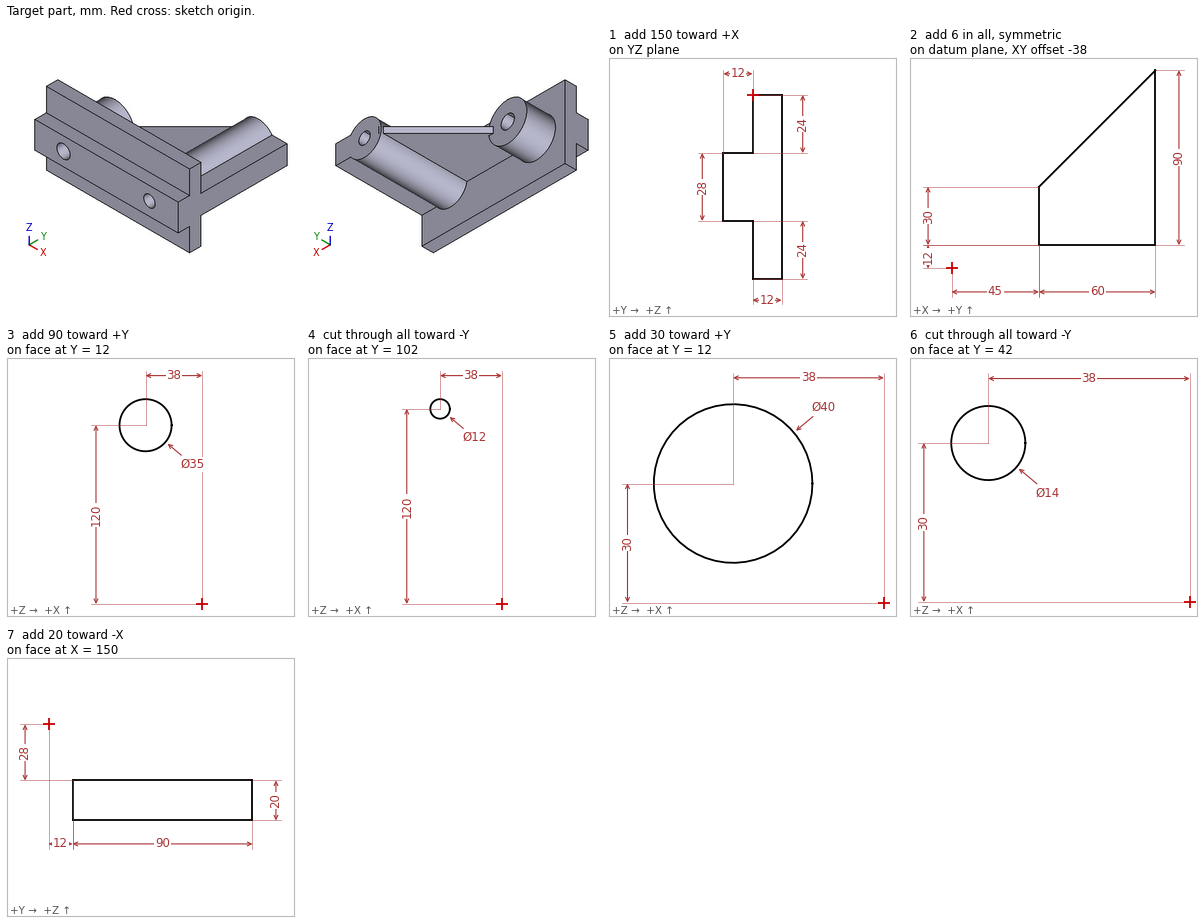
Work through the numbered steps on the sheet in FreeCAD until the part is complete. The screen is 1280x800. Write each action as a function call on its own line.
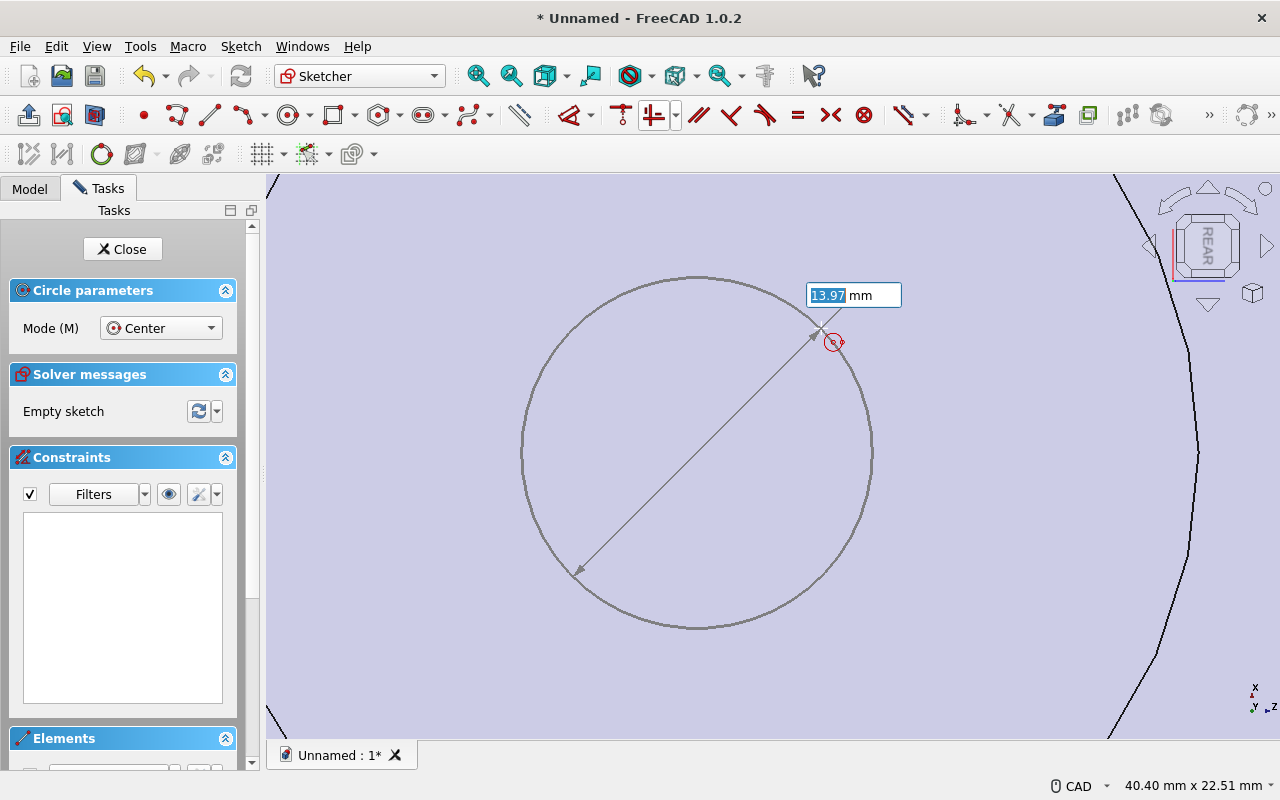
text(14)
key(Return)
key(Escape)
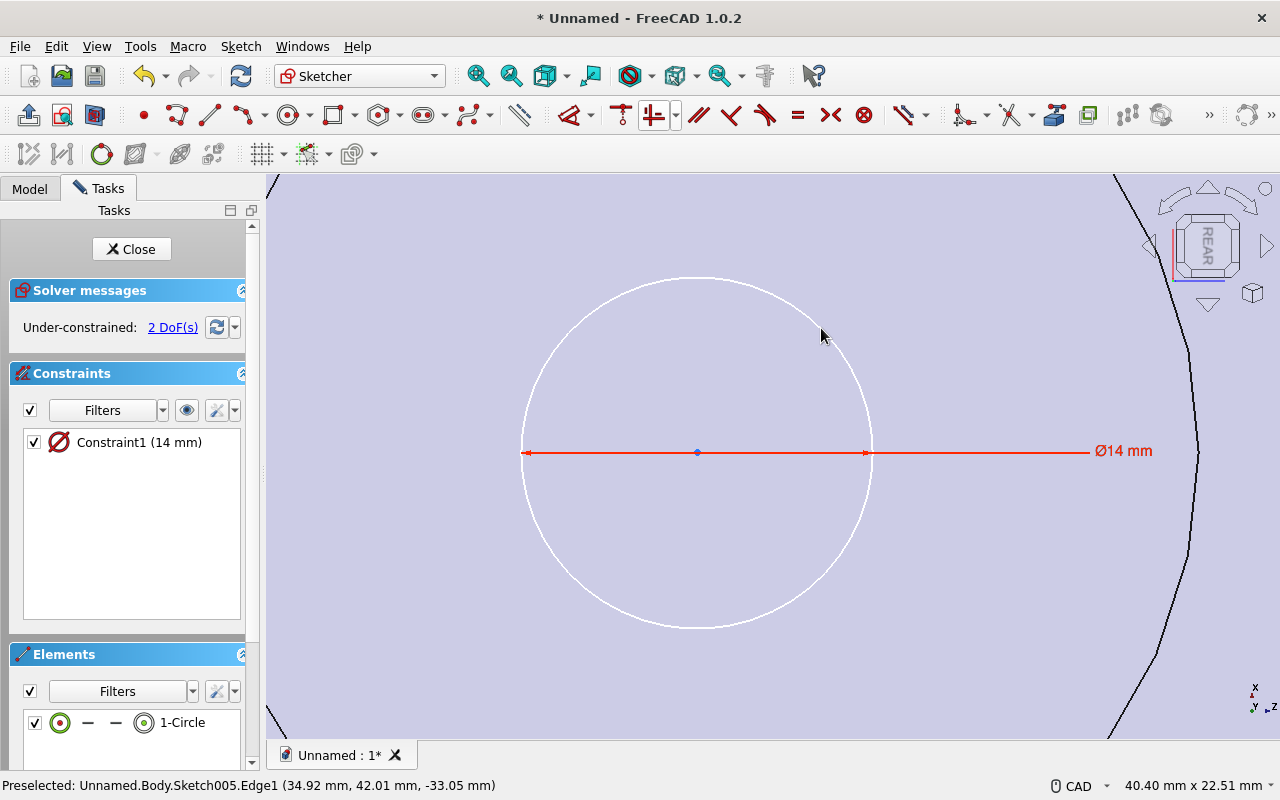
click(568, 116)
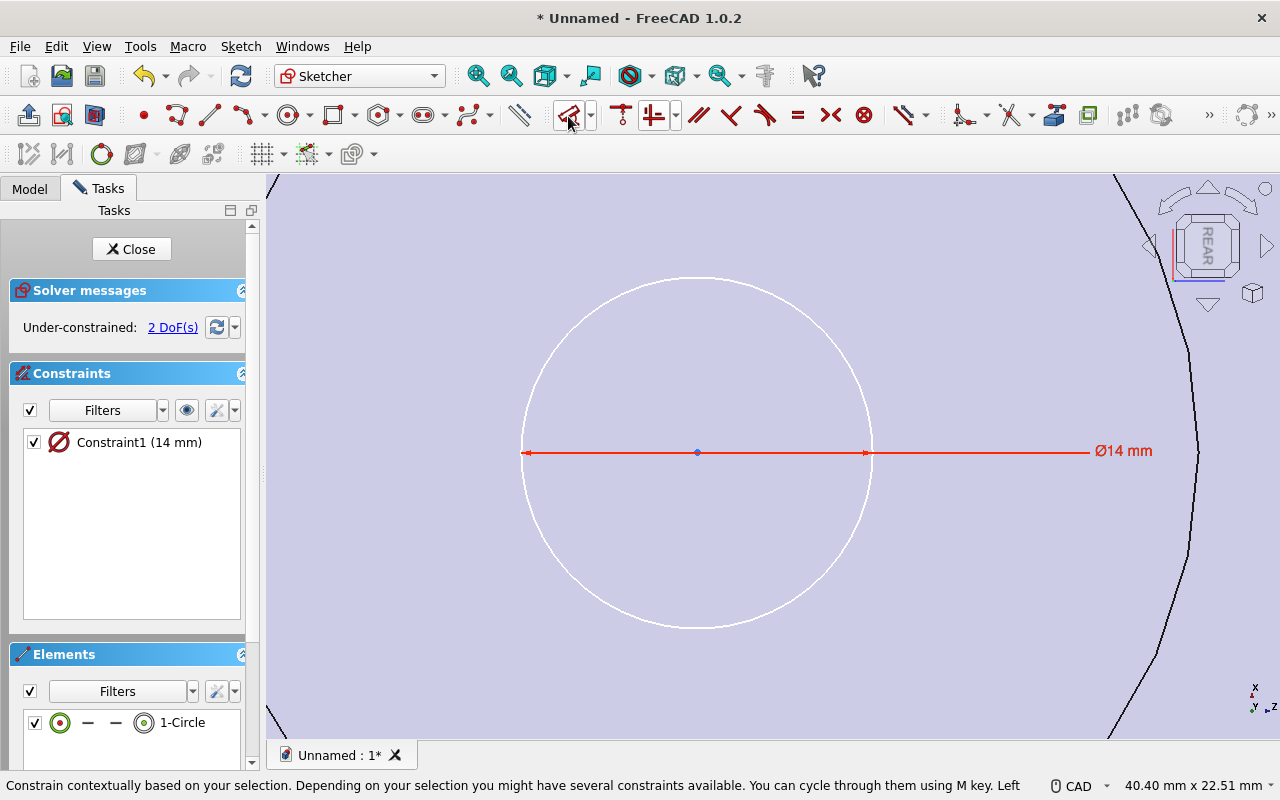
click(697, 453)
click(906, 419)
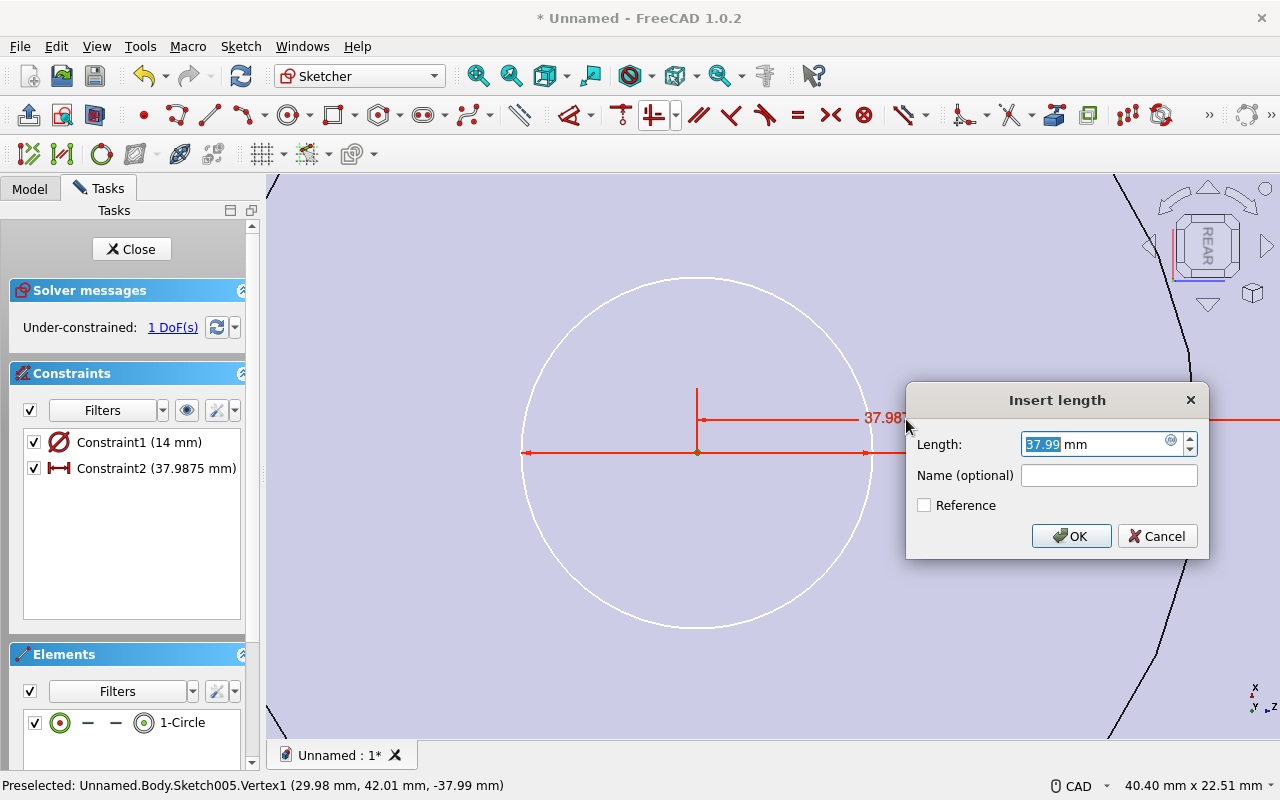
text(38)
key(Return)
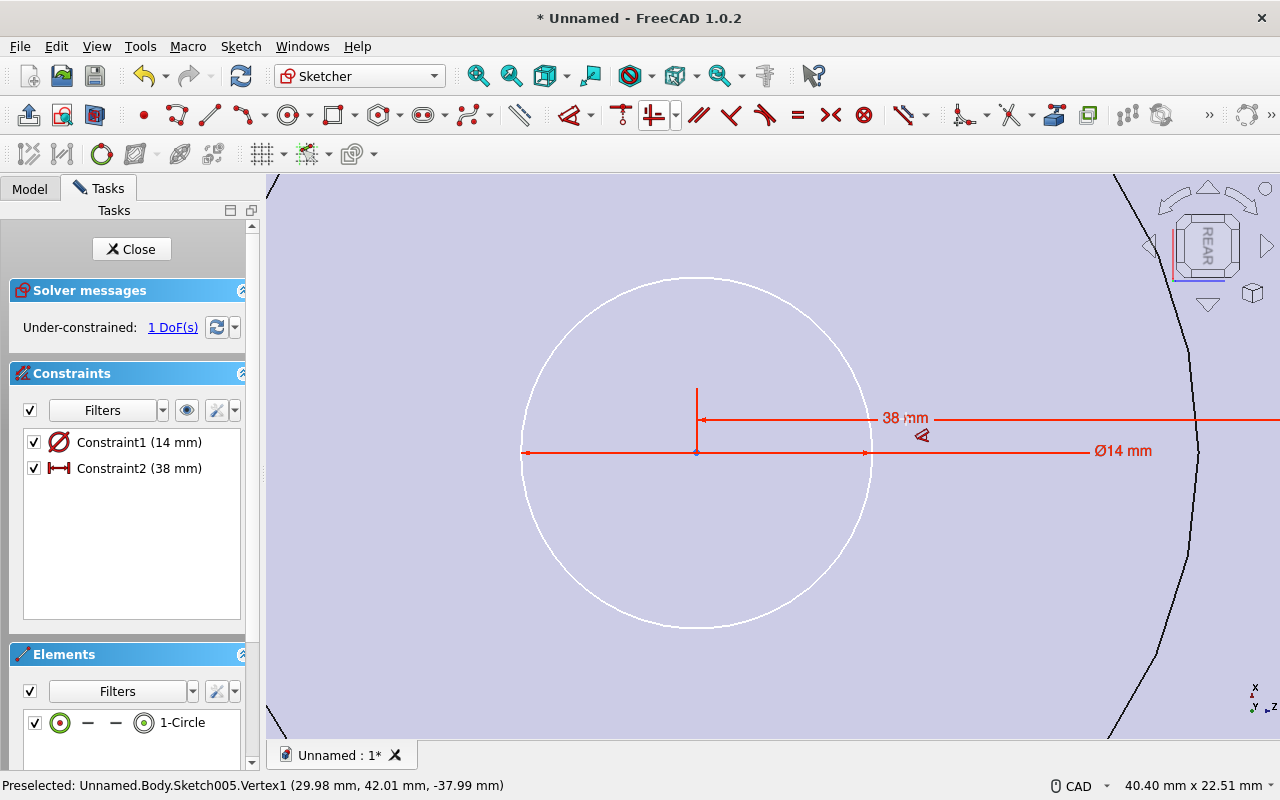
click(697, 453)
click(663, 582)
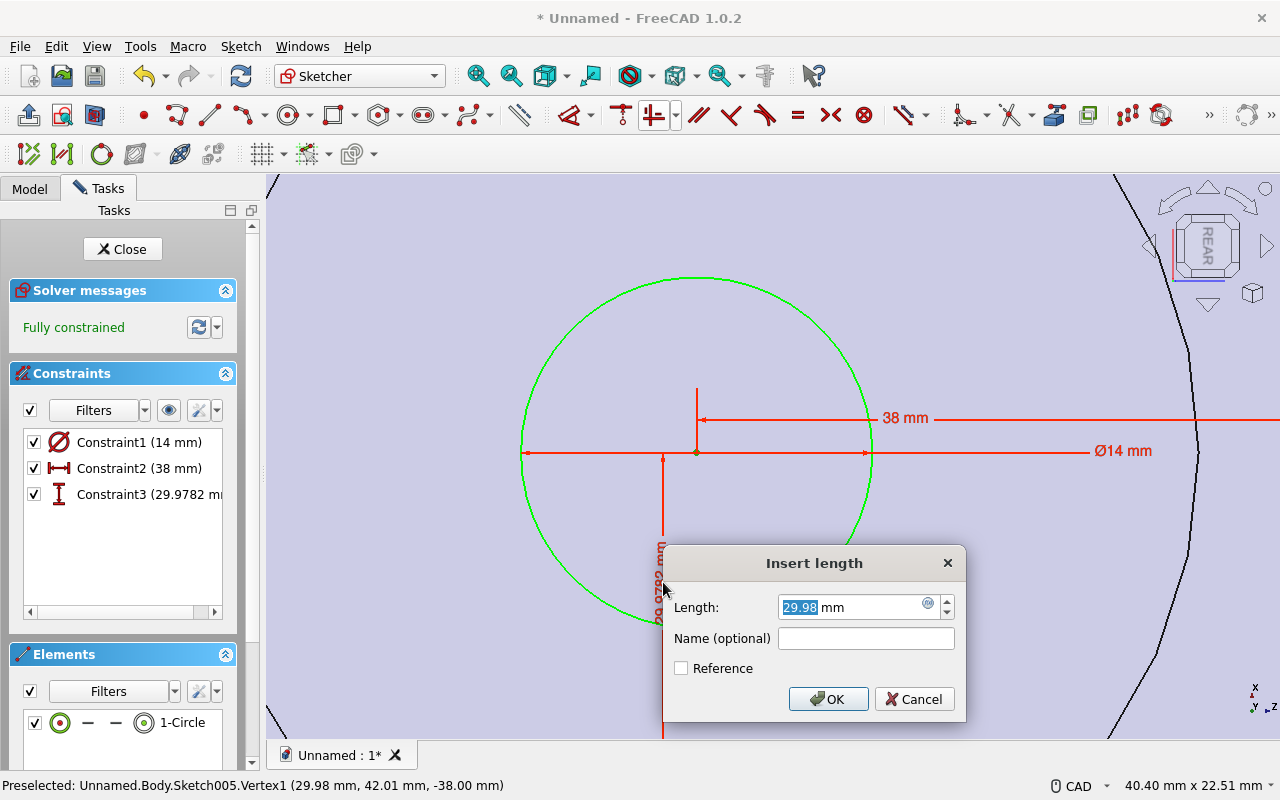
text(30)
key(Return)
key(Escape)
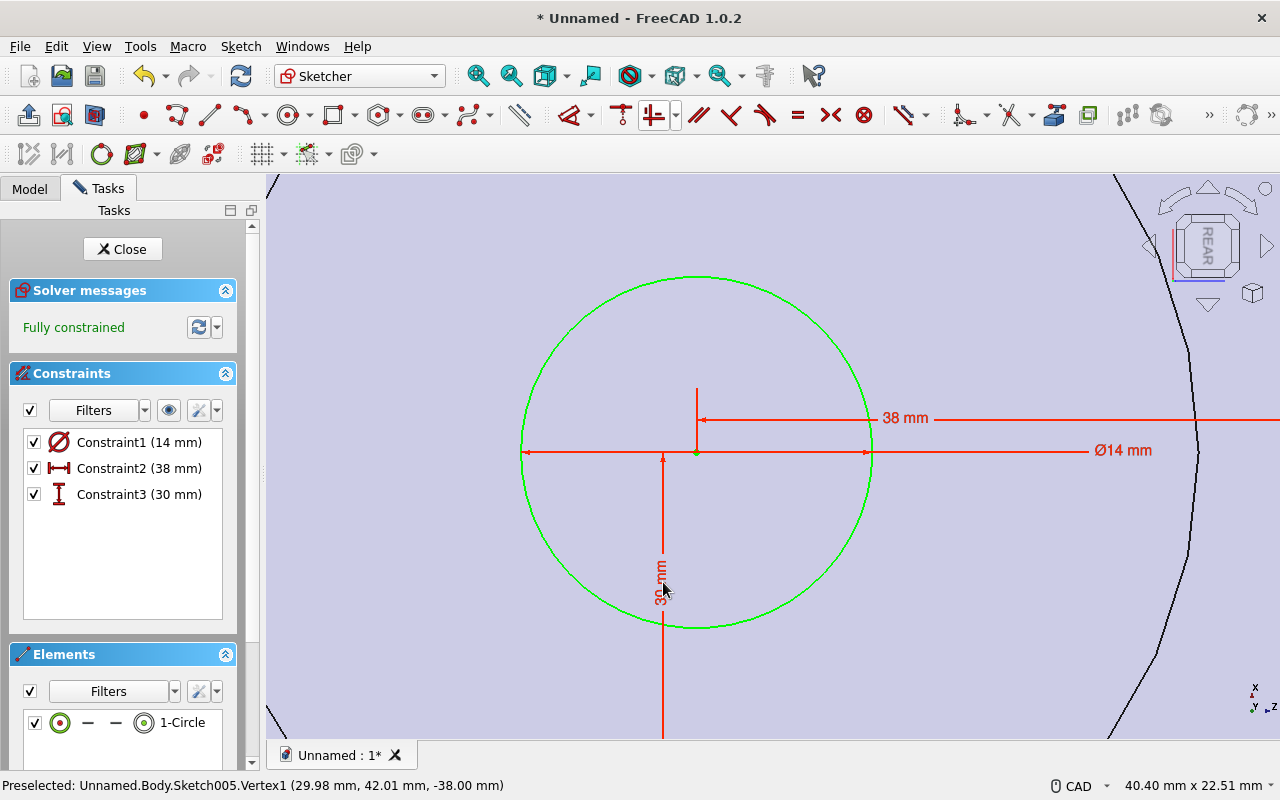
click(123, 249)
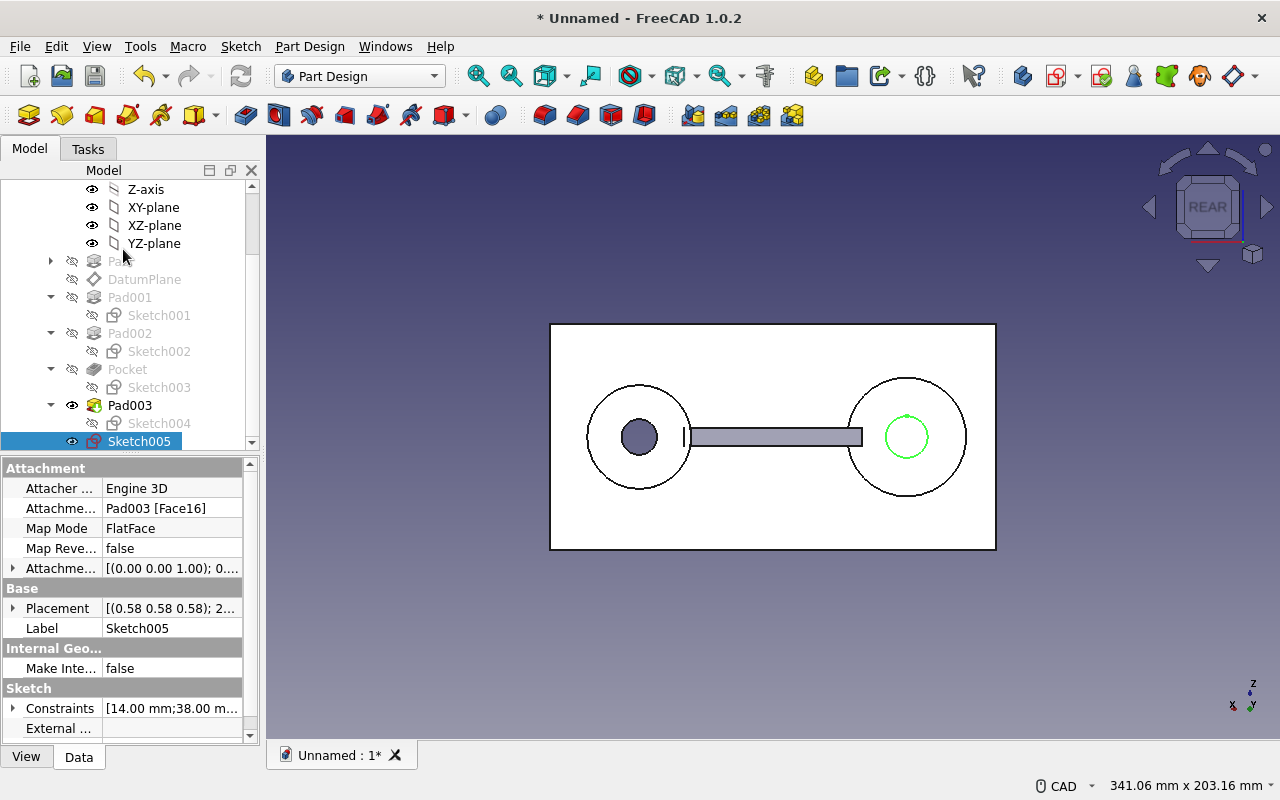
click(246, 116)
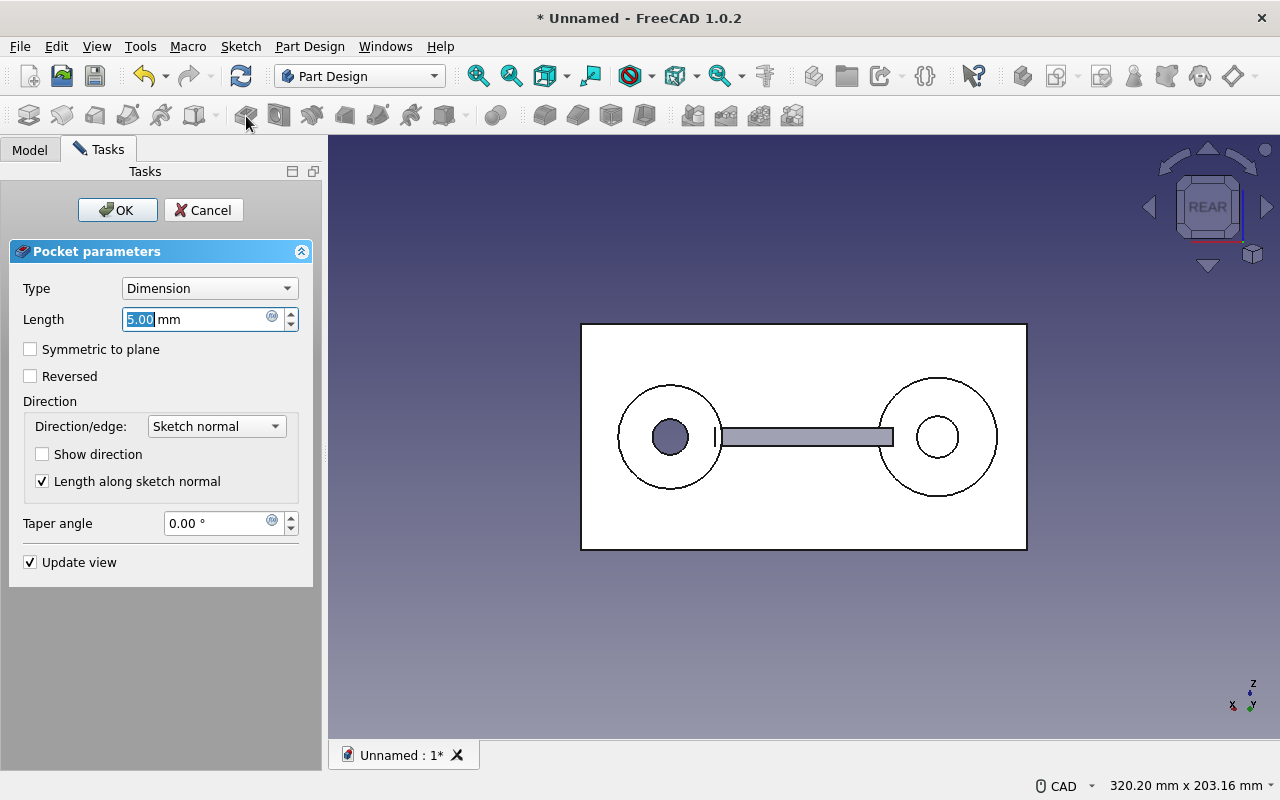
click(210, 288)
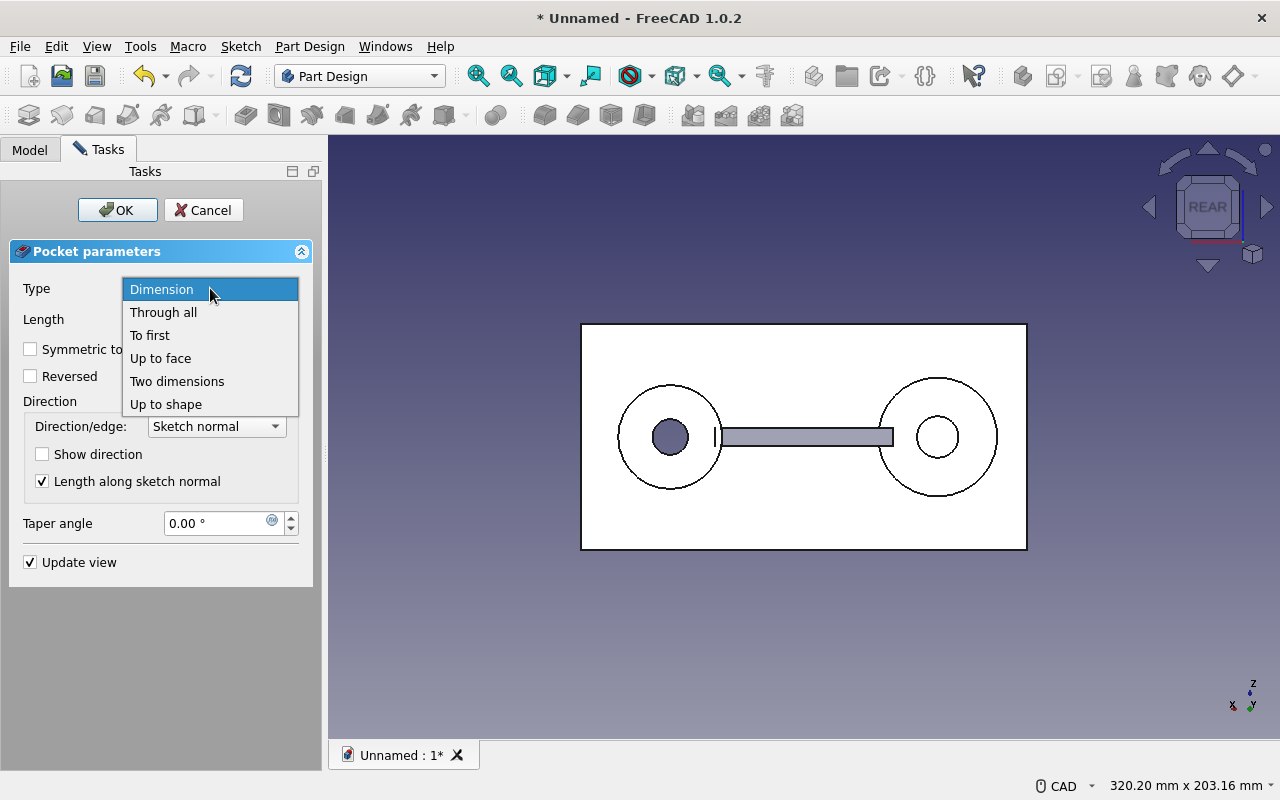
click(208, 312)